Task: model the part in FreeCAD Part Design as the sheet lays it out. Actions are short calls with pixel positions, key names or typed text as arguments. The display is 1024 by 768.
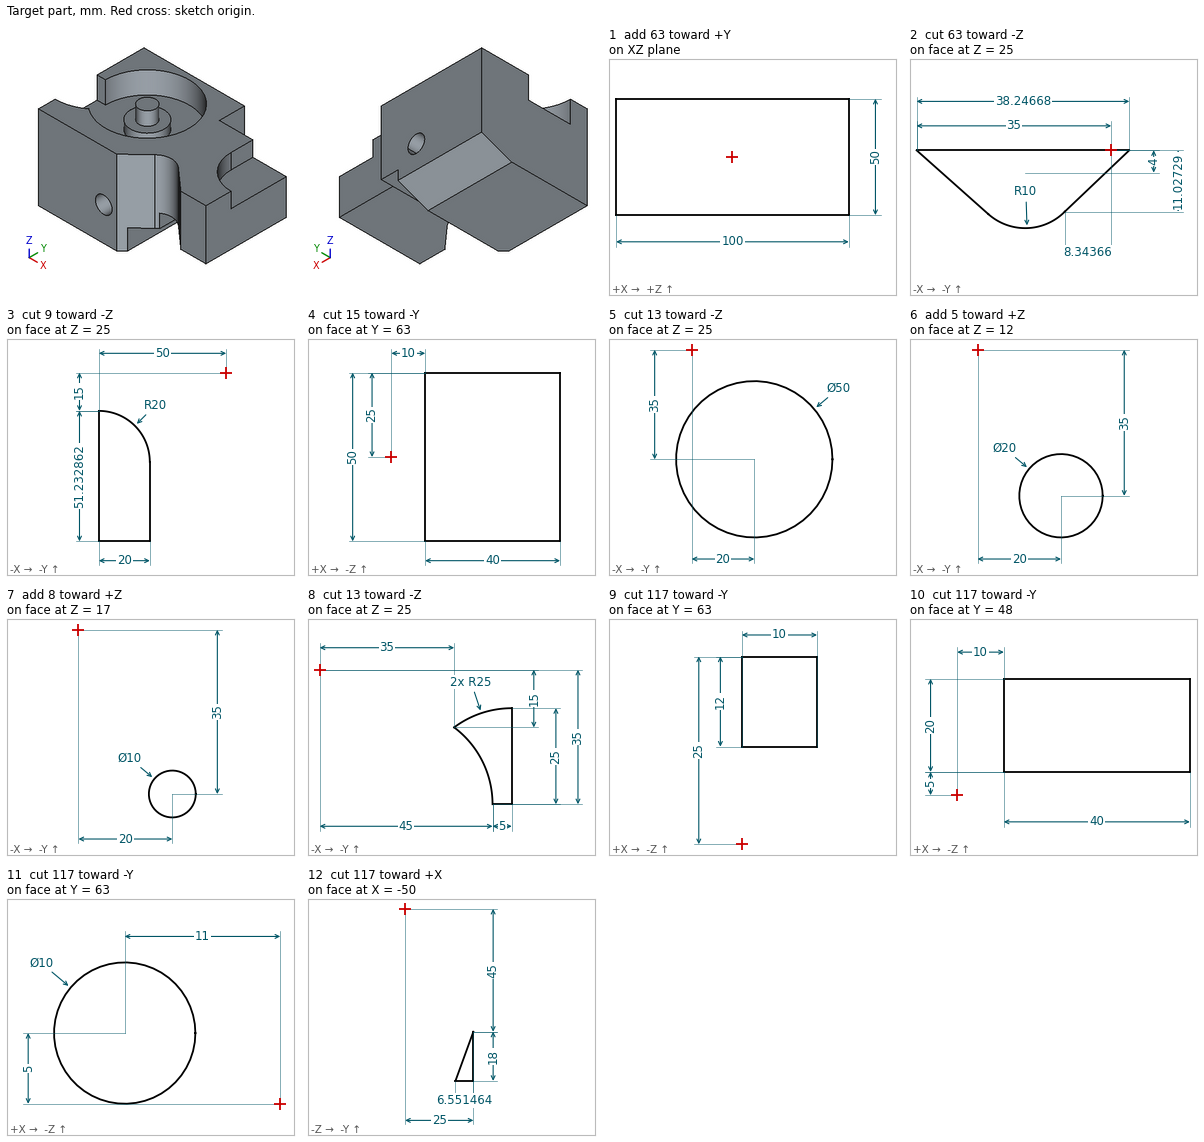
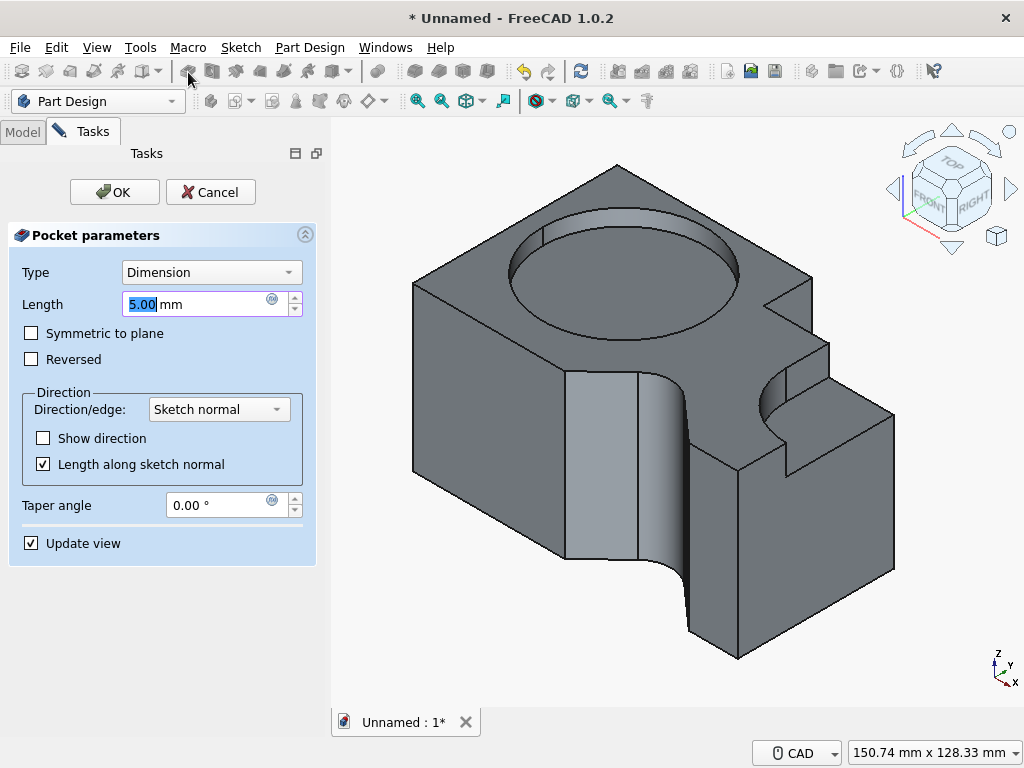
text(13)
key(Tab)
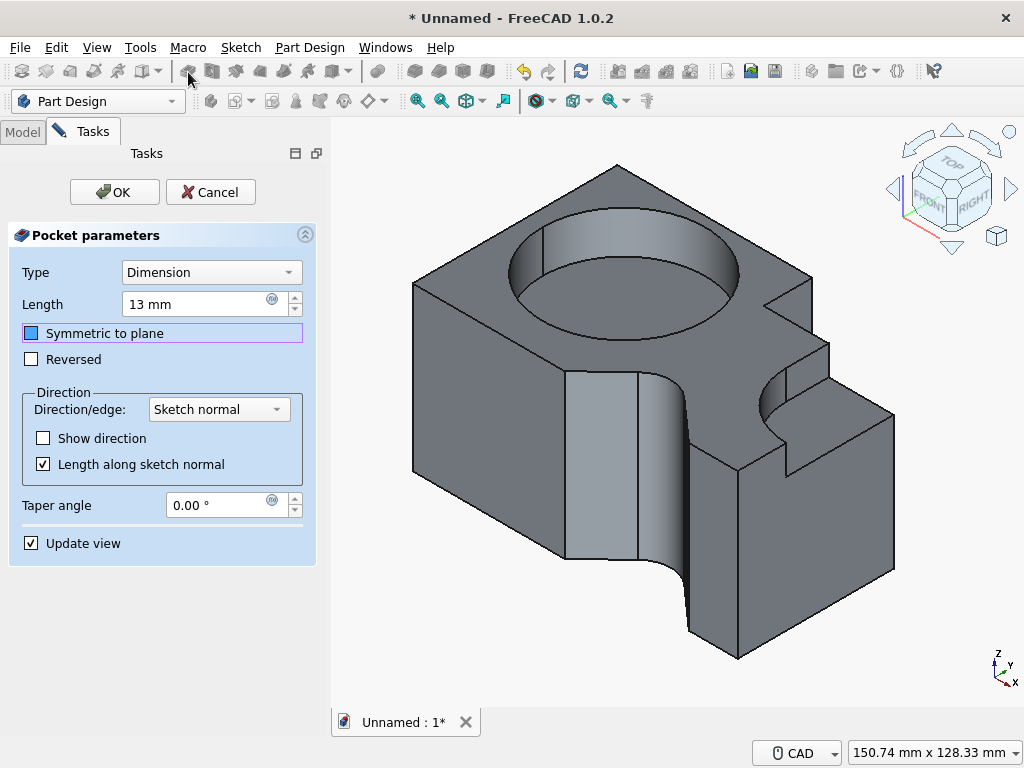
click(115, 192)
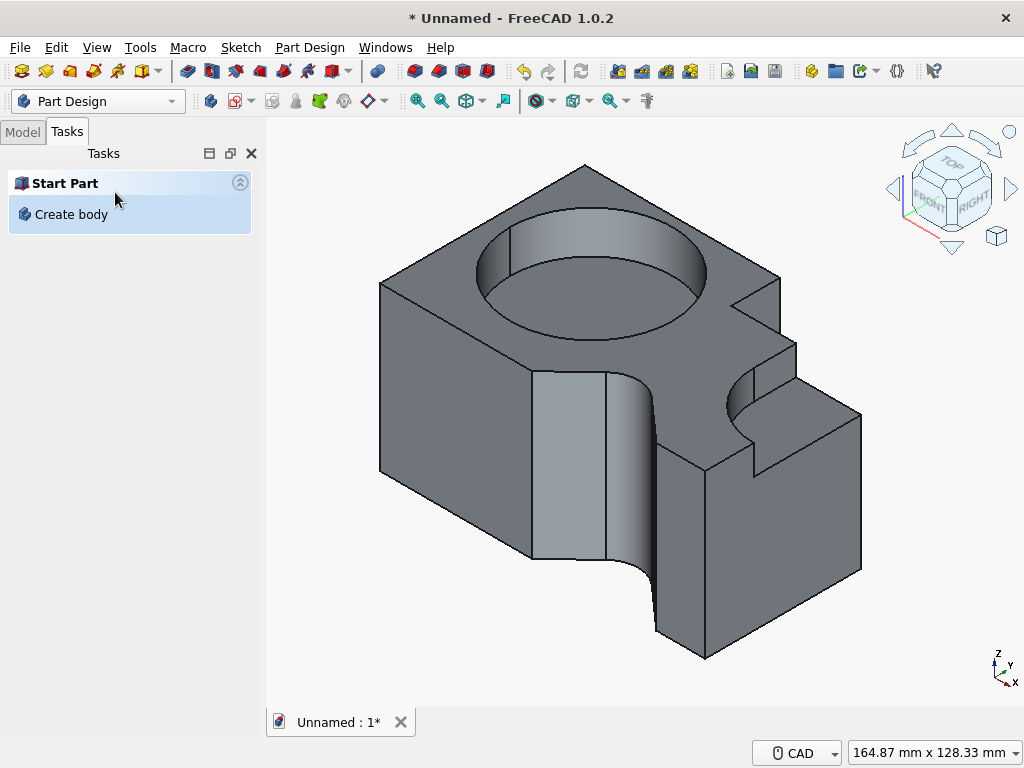
click(591, 322)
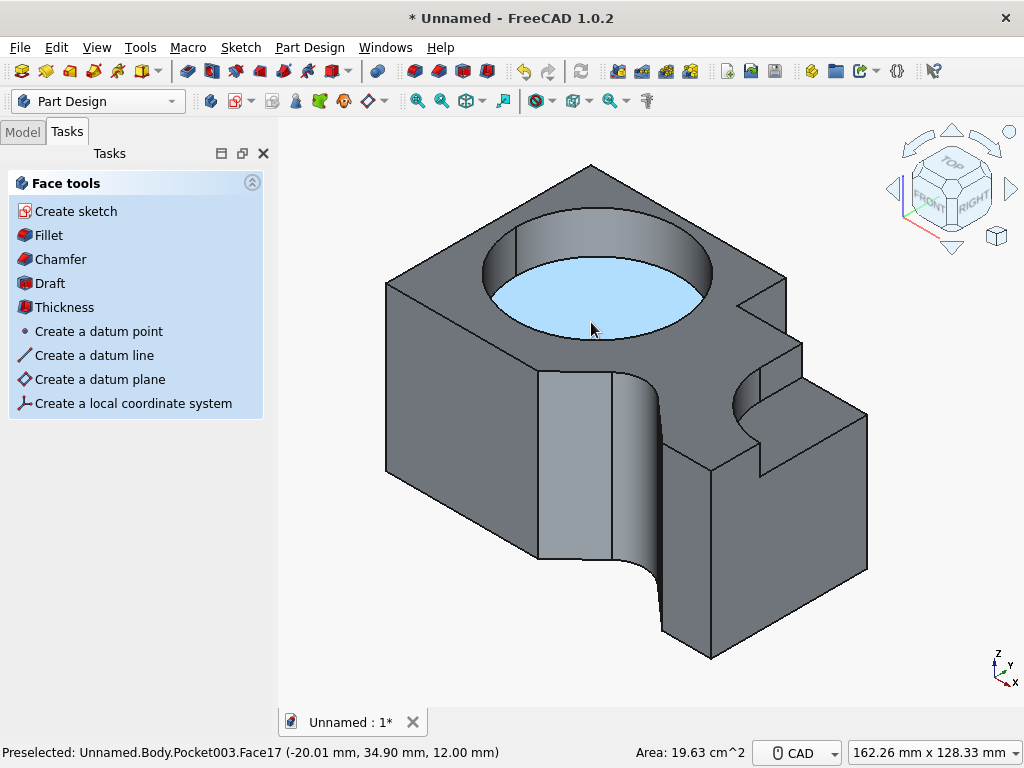
click(236, 102)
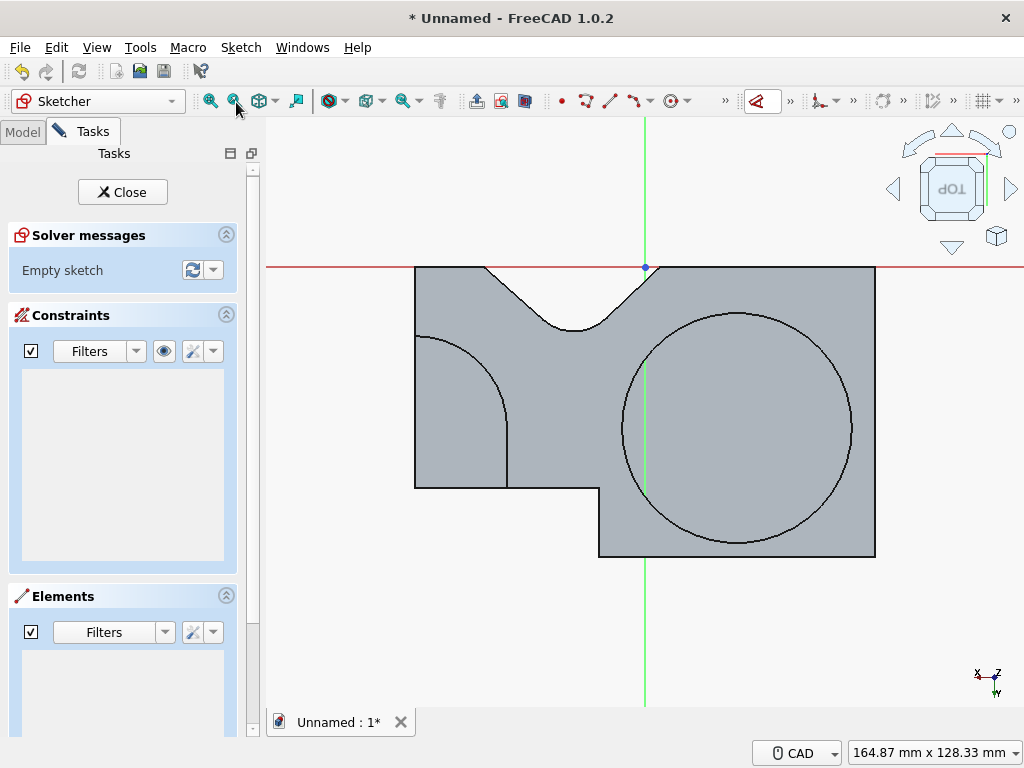
scroll(859, 320, up, 3)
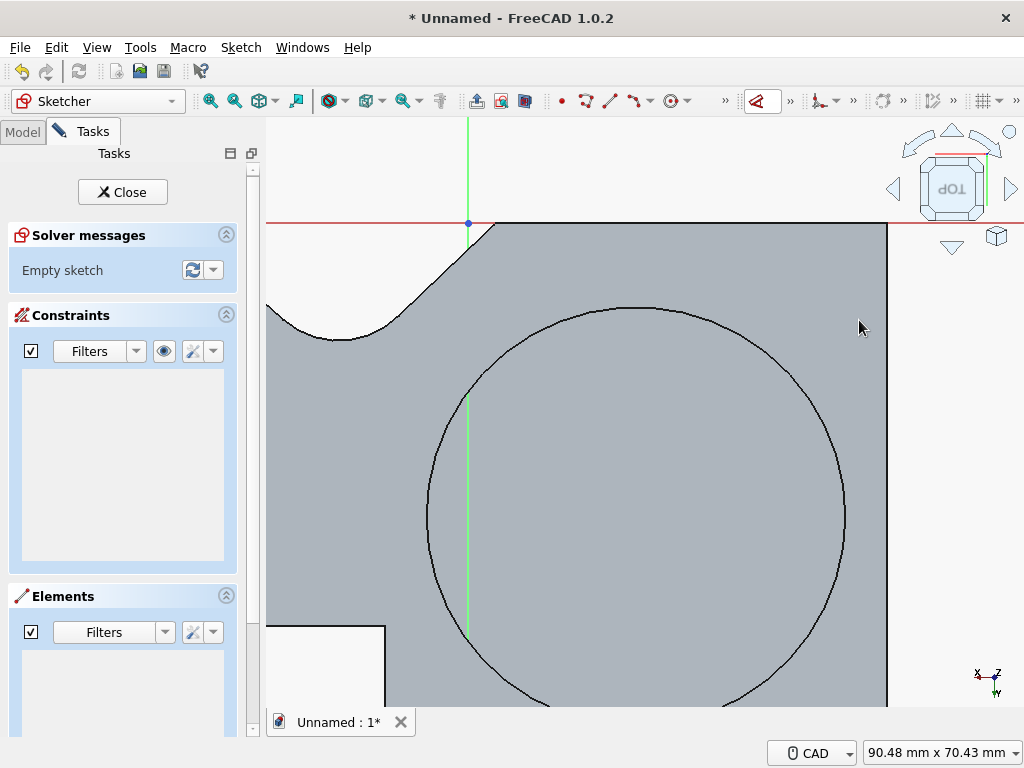
click(672, 102)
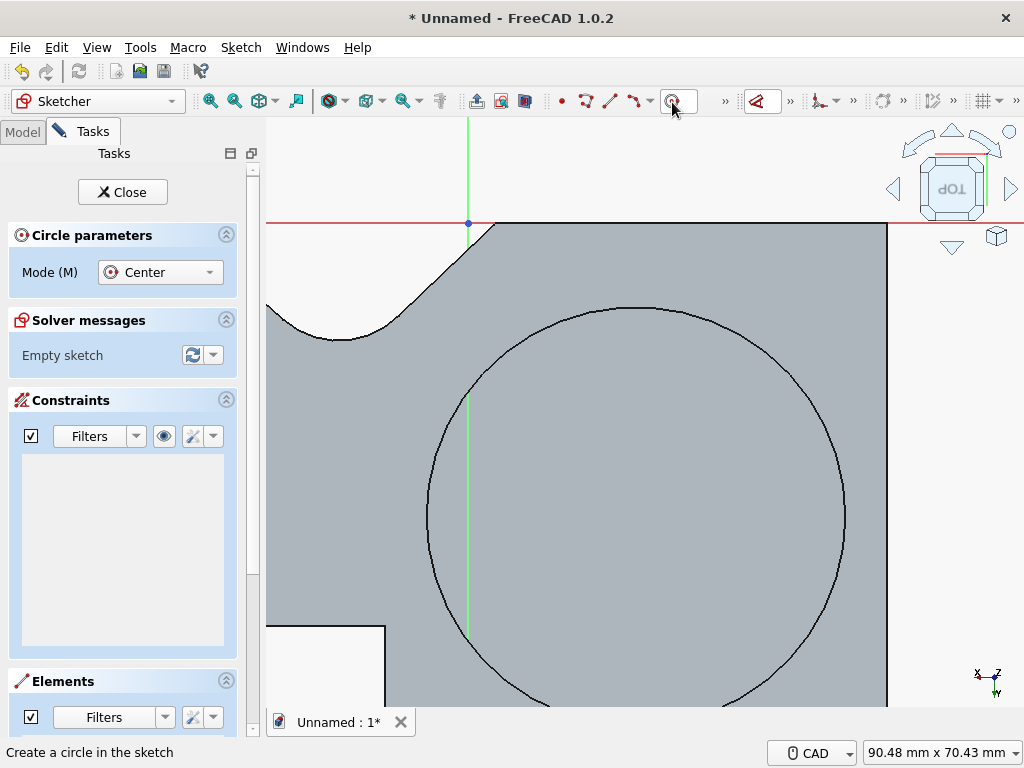
click(636, 517)
click(695, 457)
key(Escape)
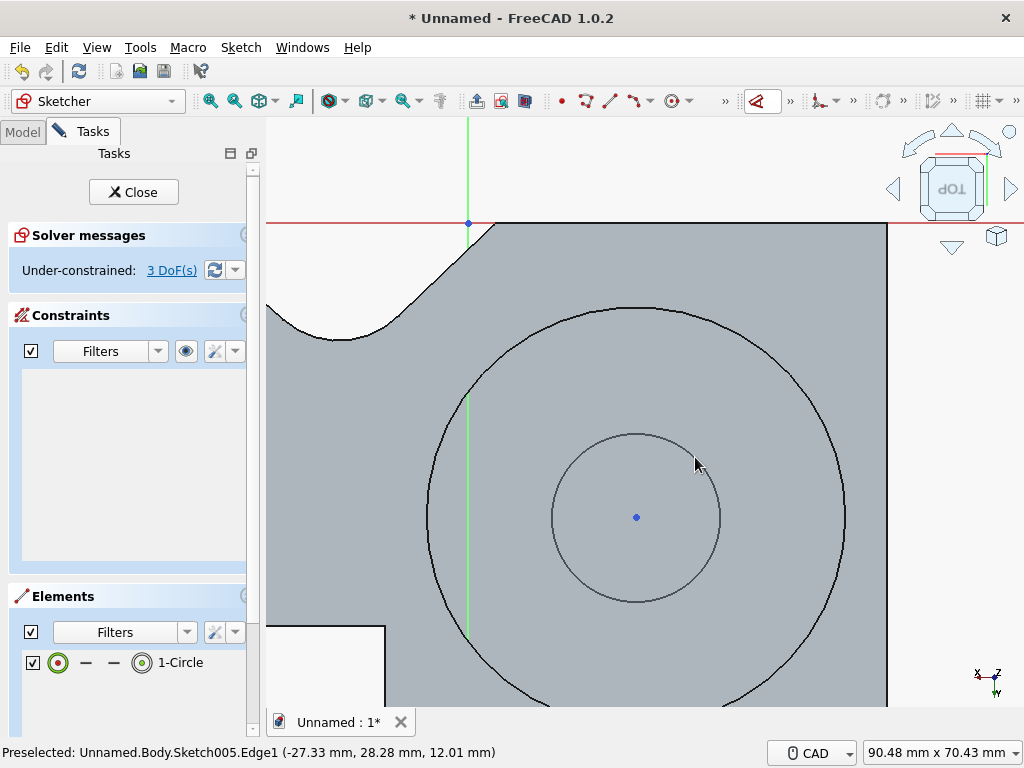
click(695, 458)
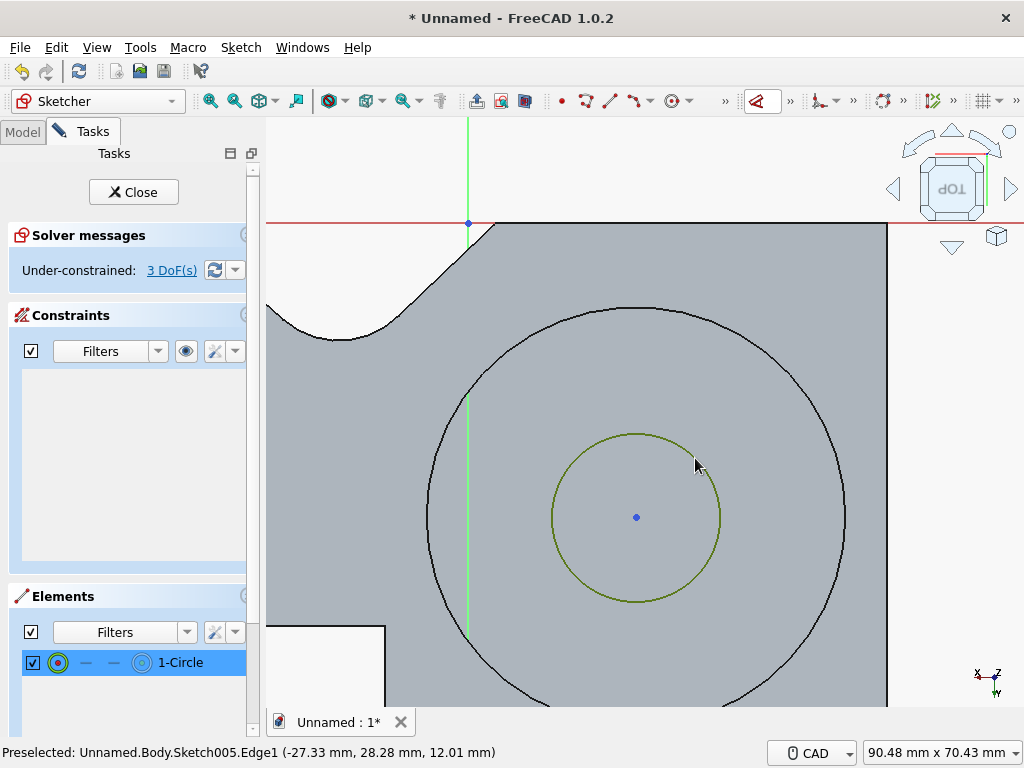
click(776, 102)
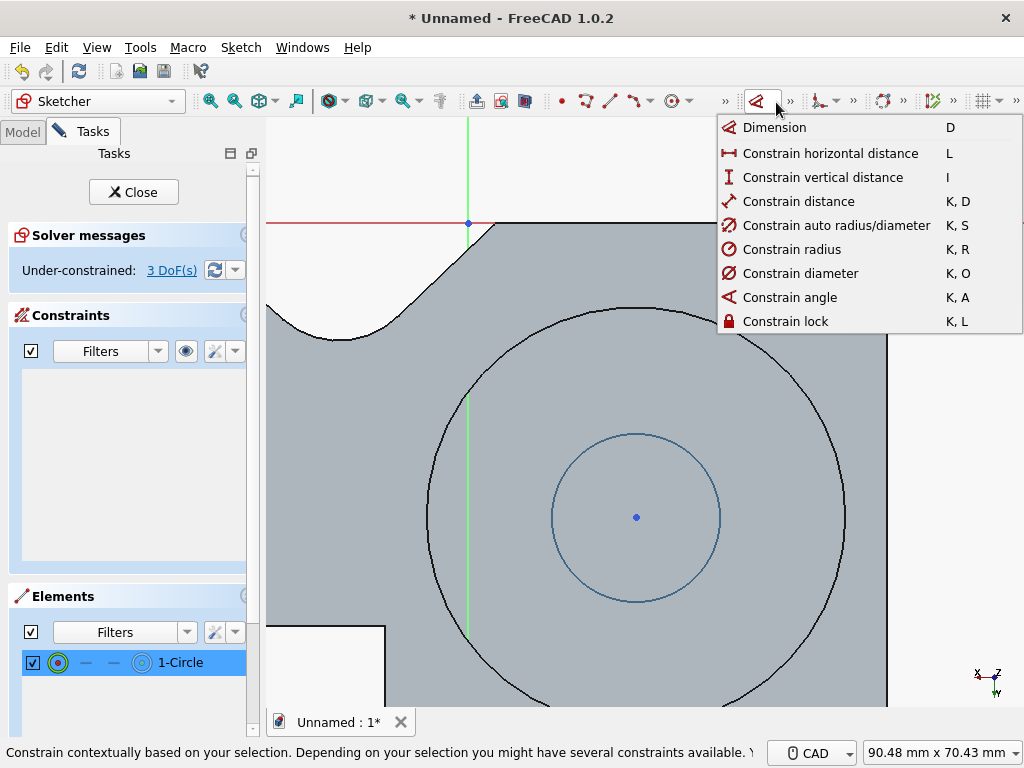
click(870, 273)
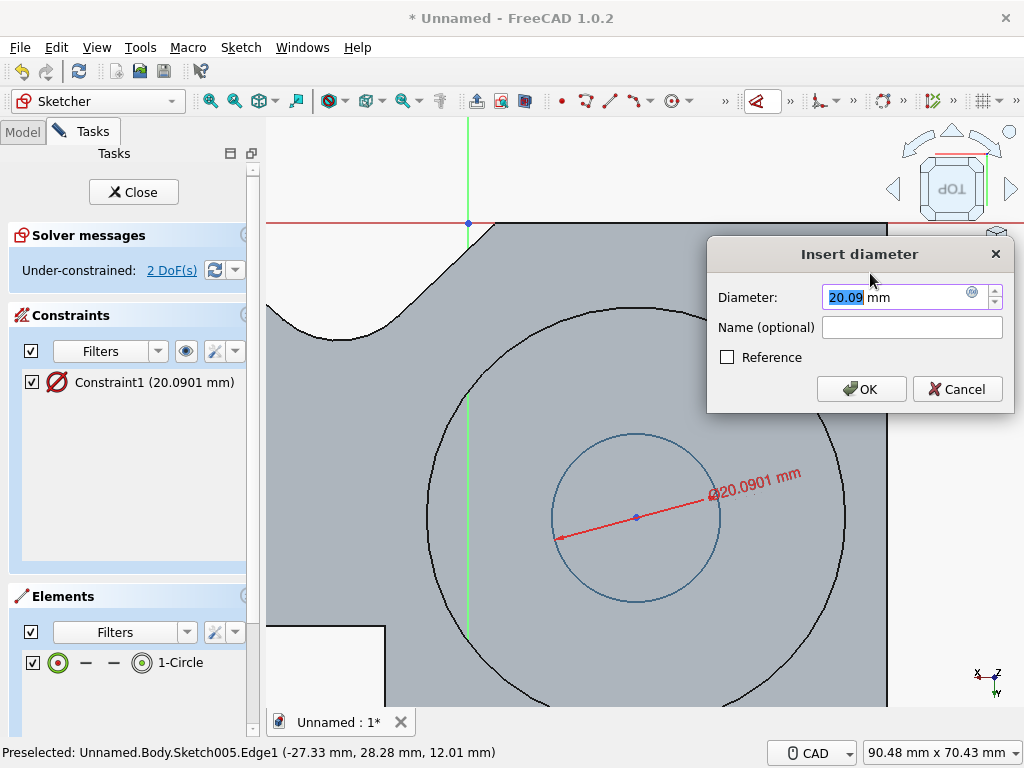
text(20)
key(Return)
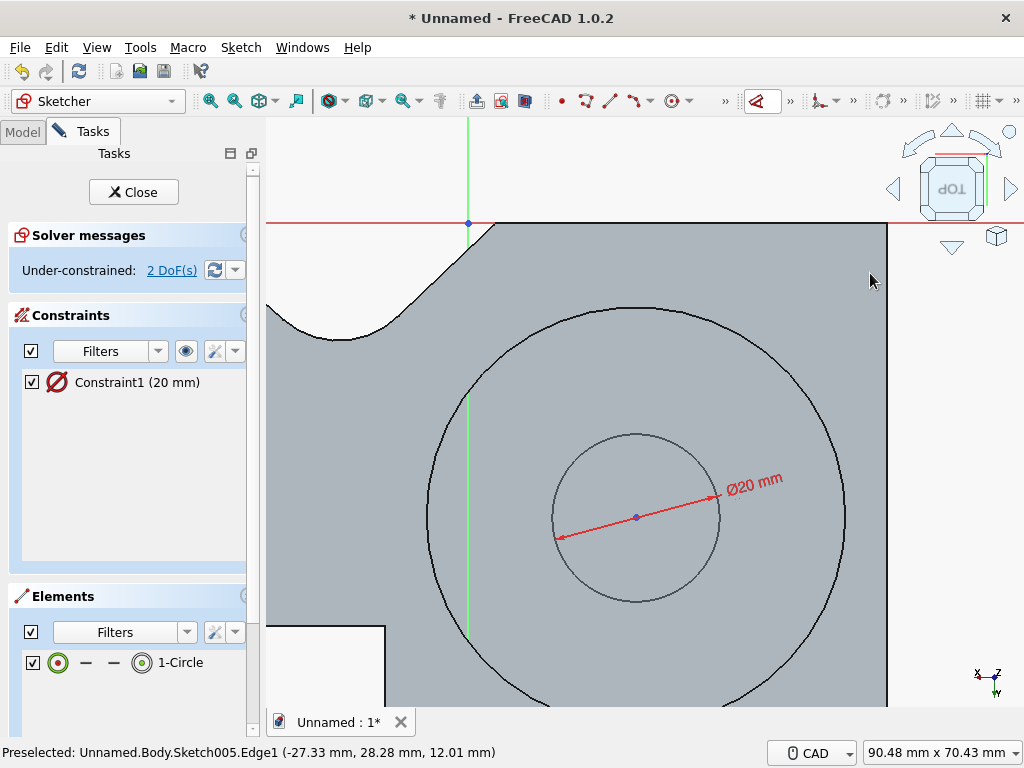
click(636, 518)